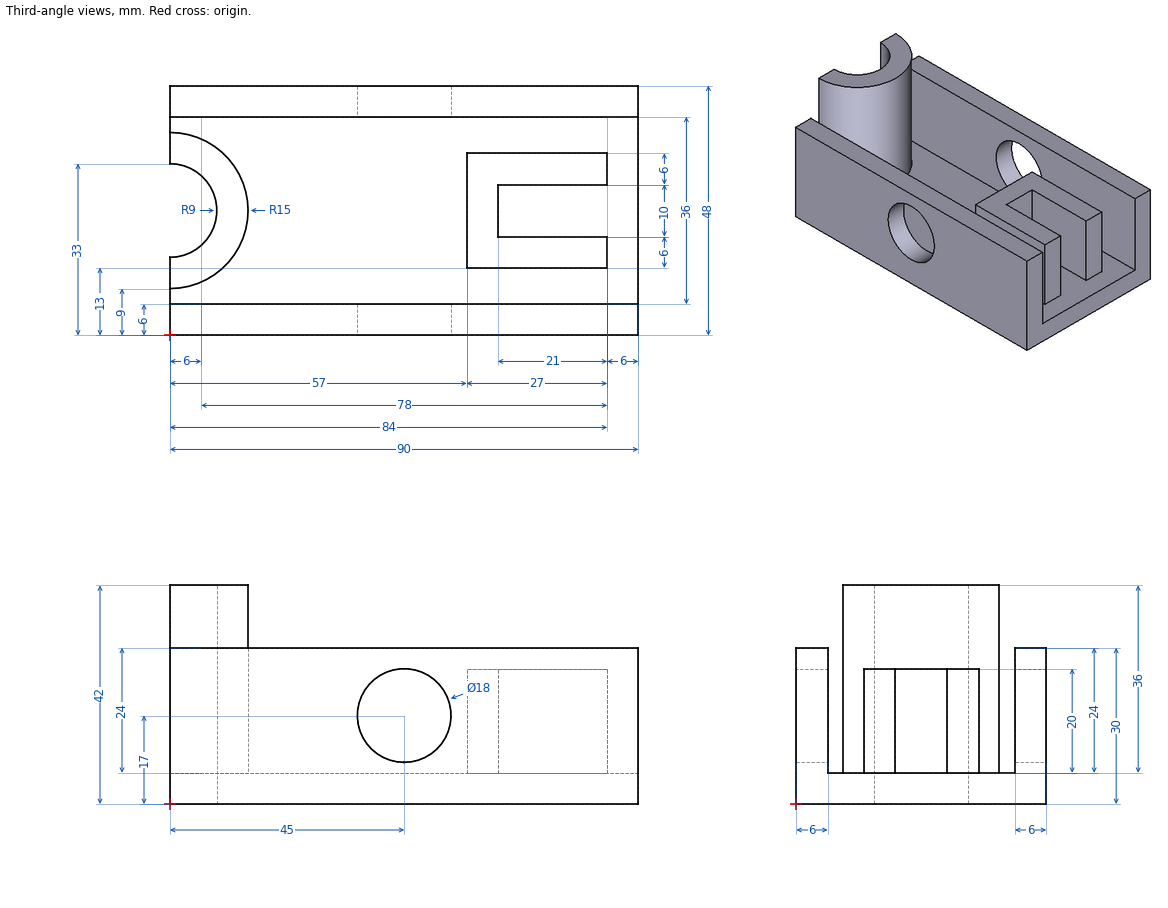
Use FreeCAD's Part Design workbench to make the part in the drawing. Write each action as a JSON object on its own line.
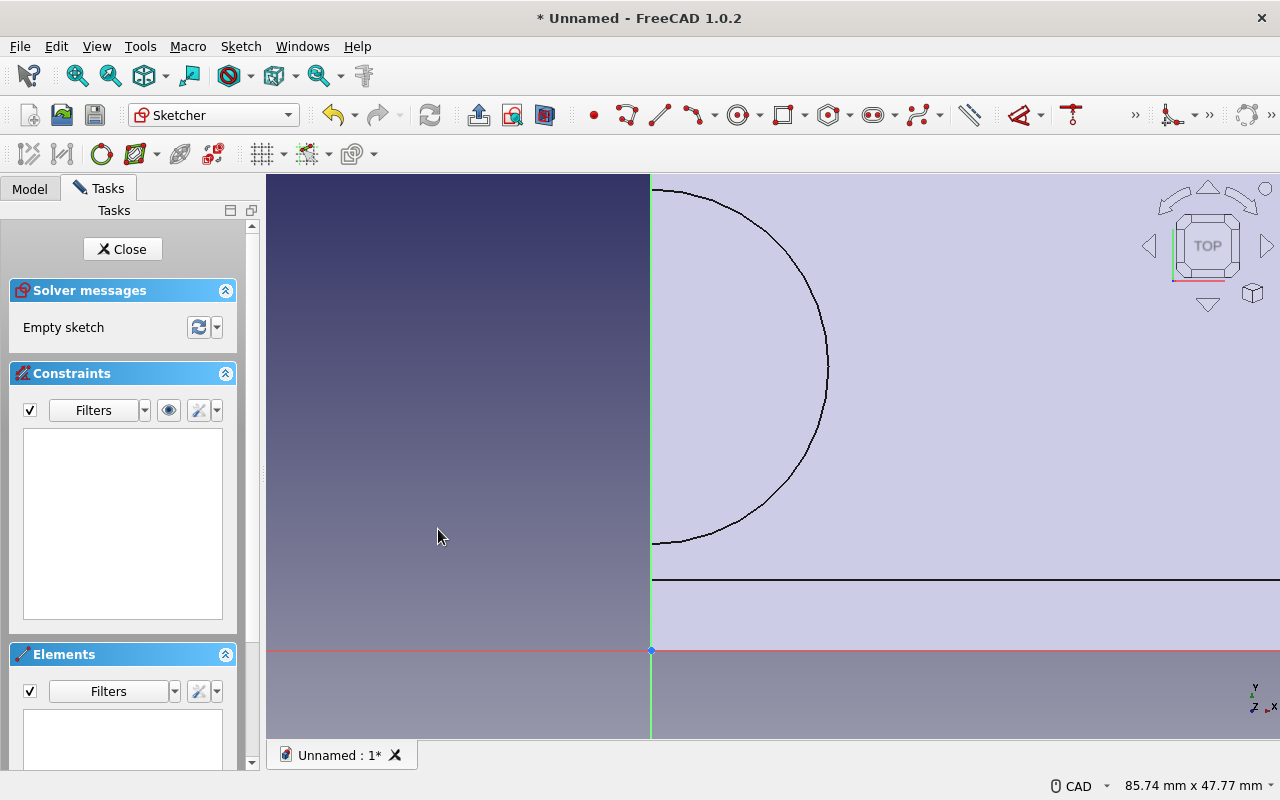
{"action": "left_click", "coordinate": [660, 116]}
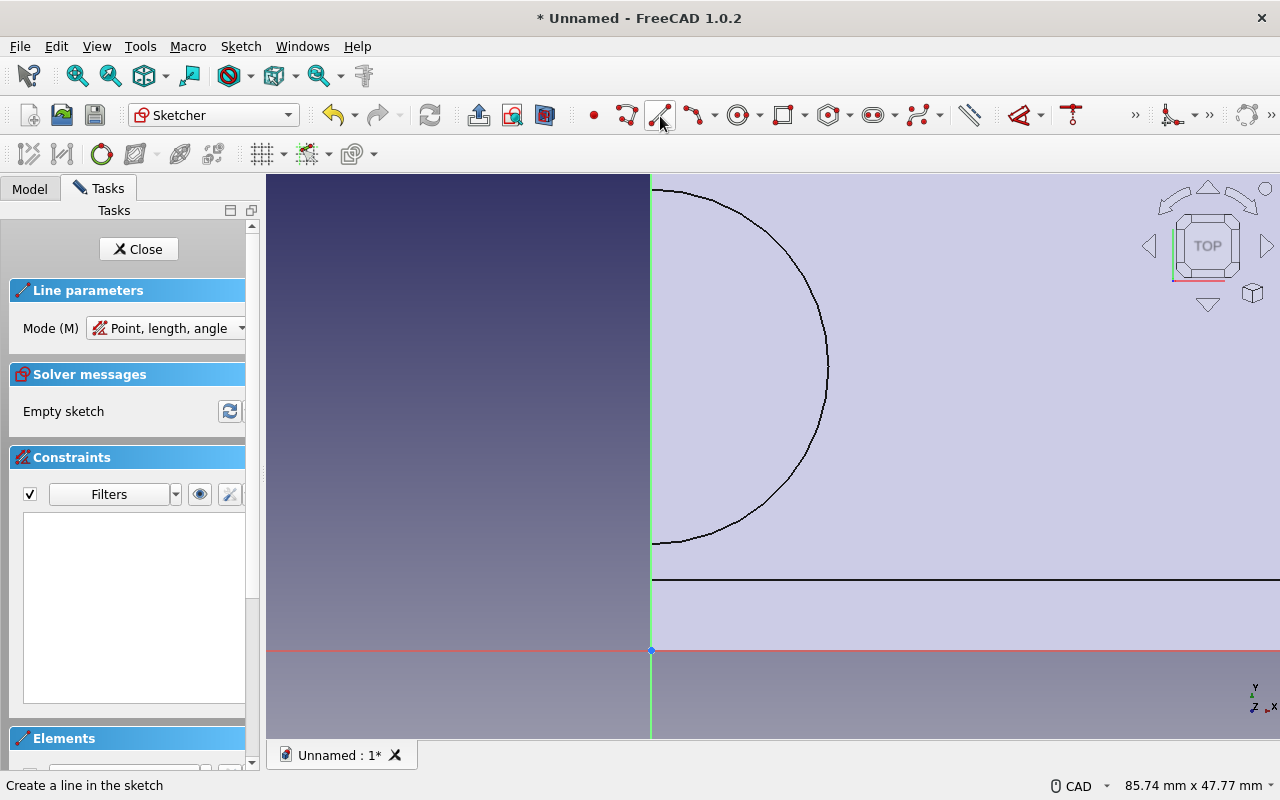
{"action": "left_click", "coordinate": [651, 260]}
{"action": "left_click", "coordinate": [660, 473]}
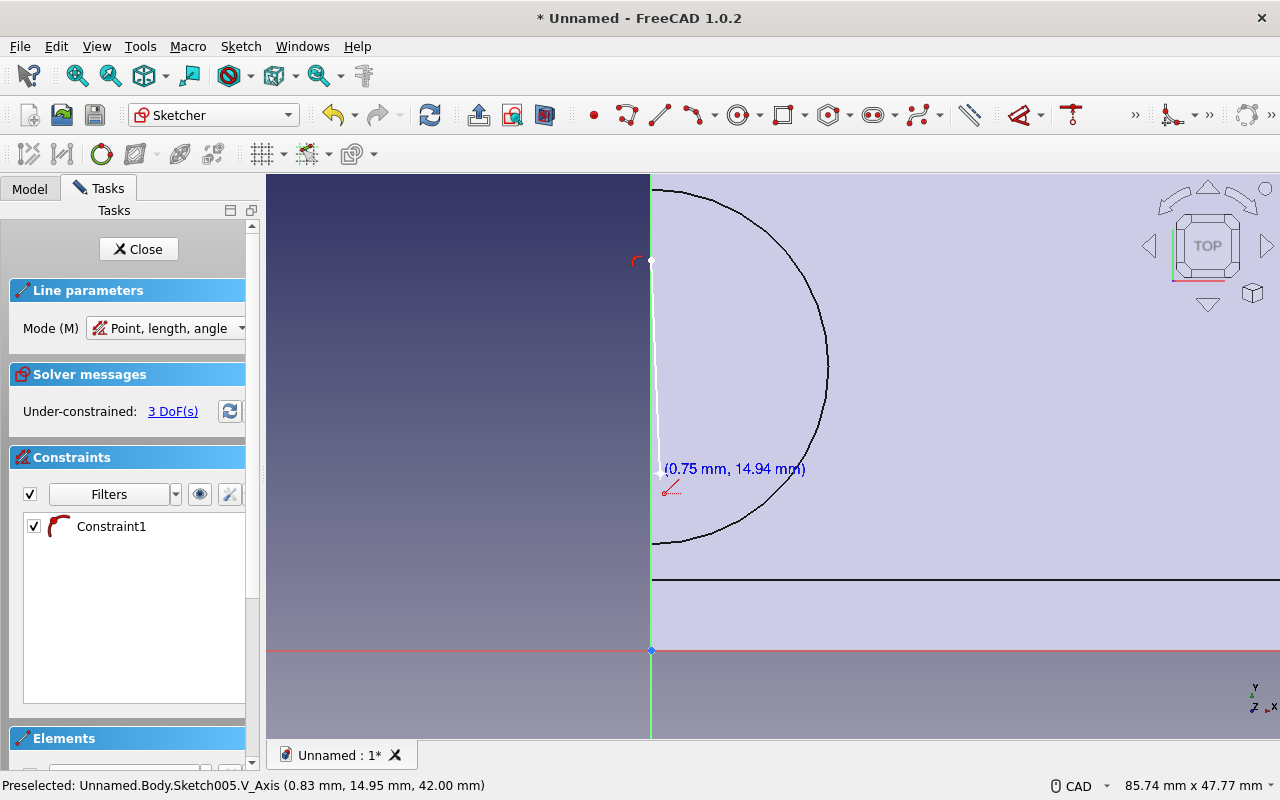
{"action": "key", "text": "g 3 a"}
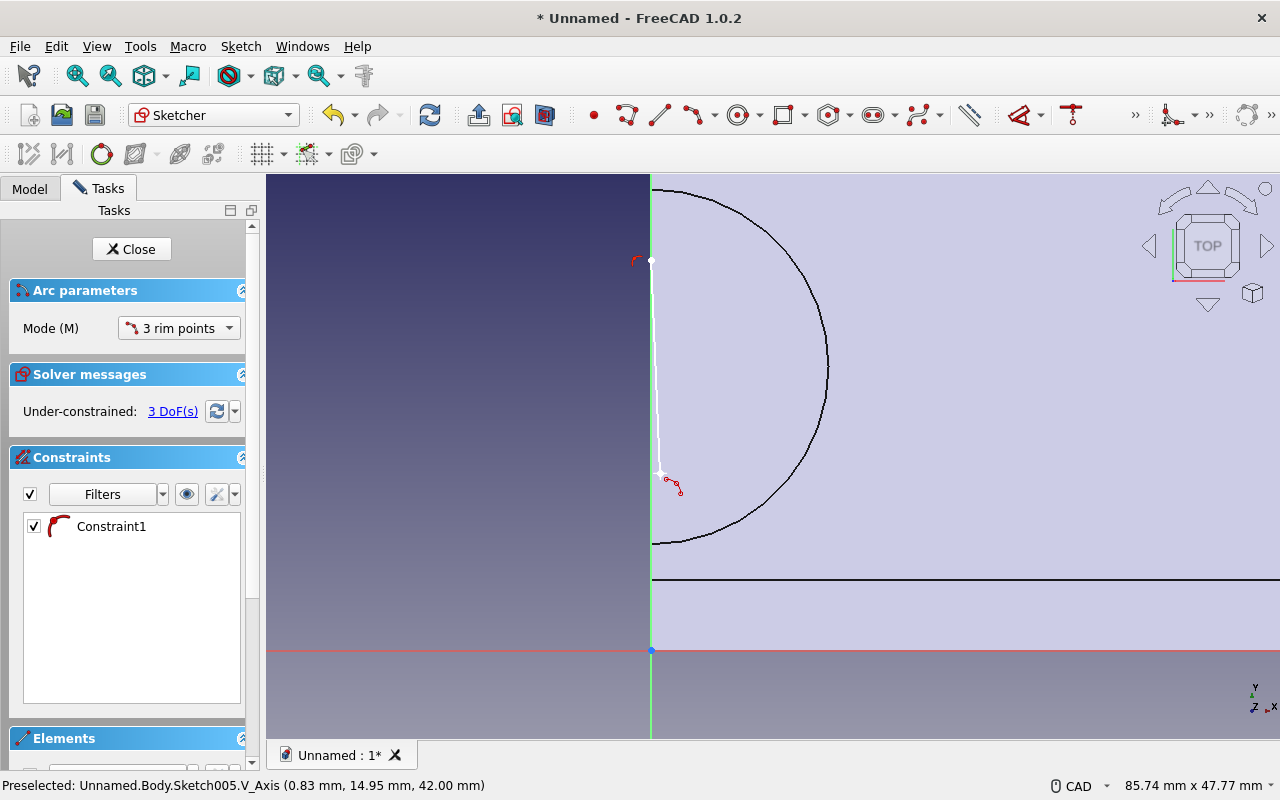
{"action": "left_click", "coordinate": [660, 474]}
{"action": "left_click", "coordinate": [651, 261]}
{"action": "left_click", "coordinate": [758, 367]}
{"action": "key", "text": "Escape"}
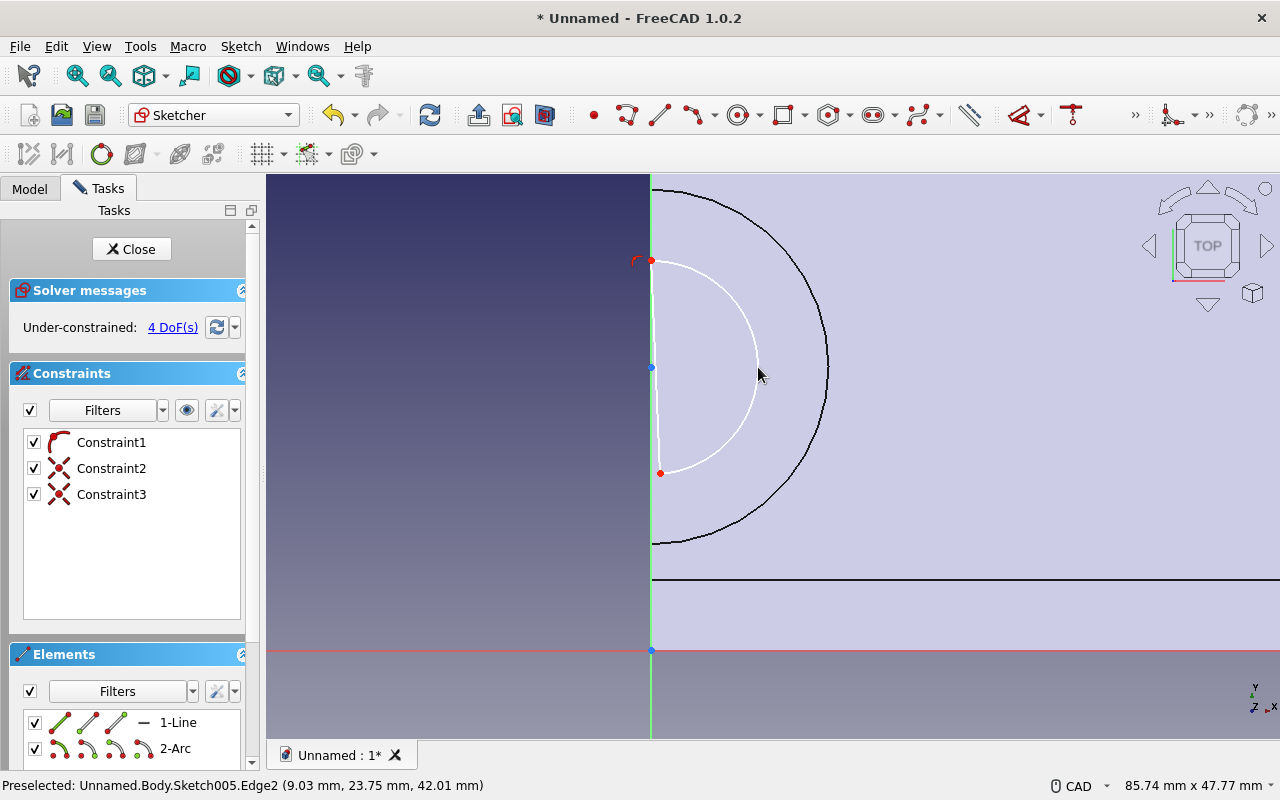
{"action": "left_click", "coordinate": [654, 325]}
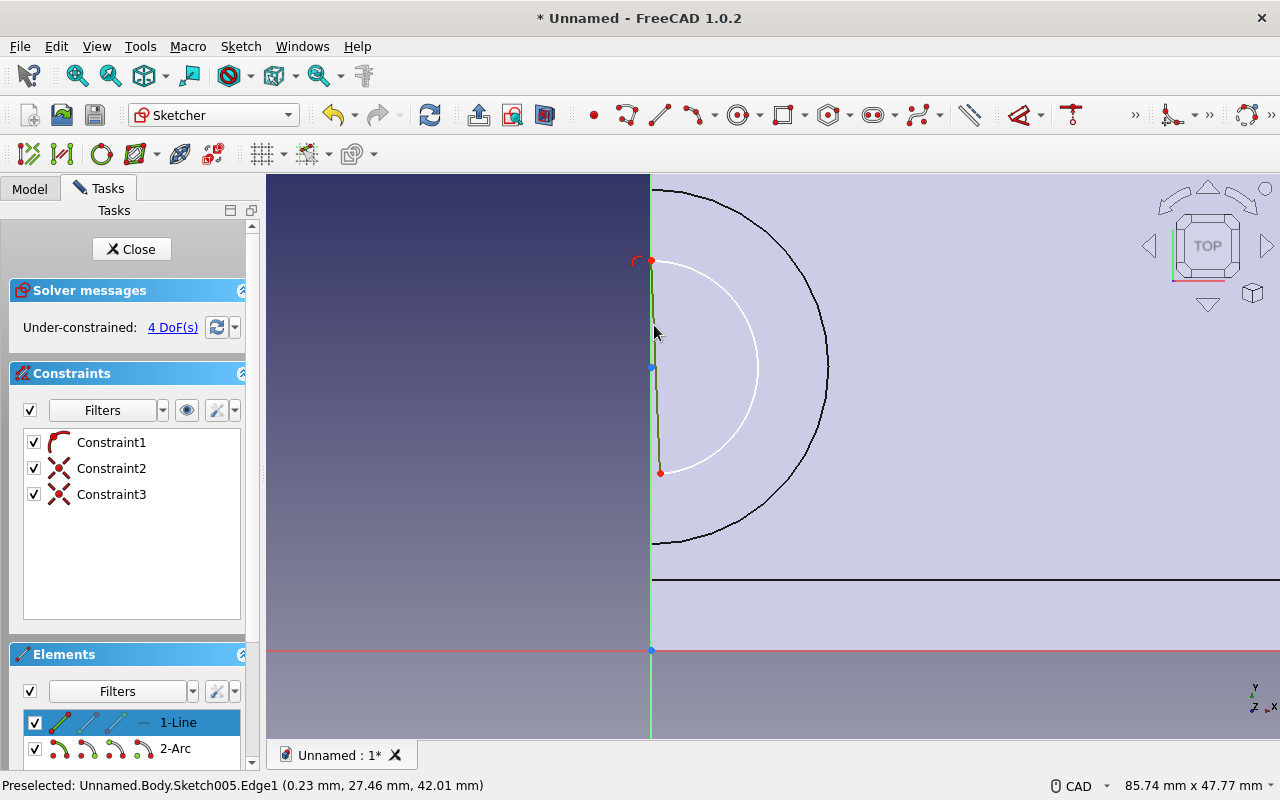
{"action": "key", "text": "v"}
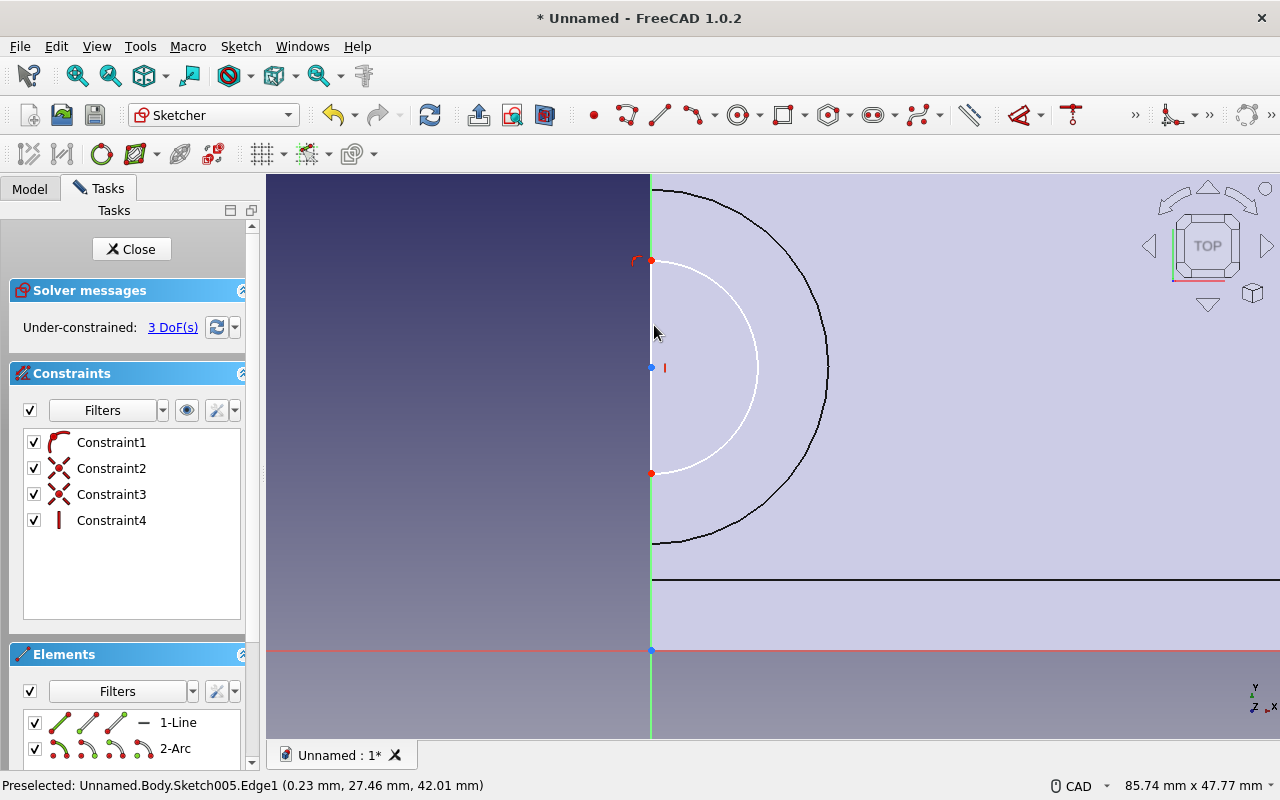
{"action": "left_click", "coordinate": [651, 368]}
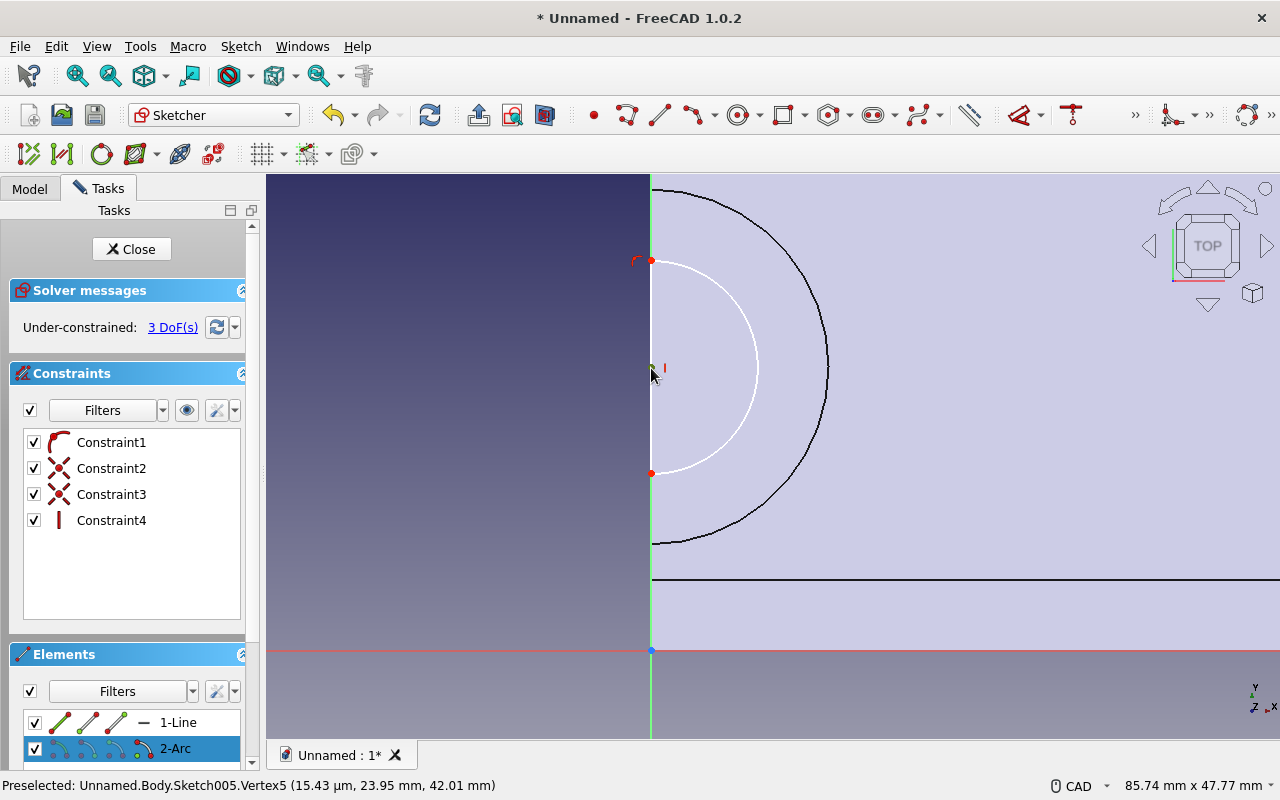
{"action": "left_click", "coordinate": [651, 602]}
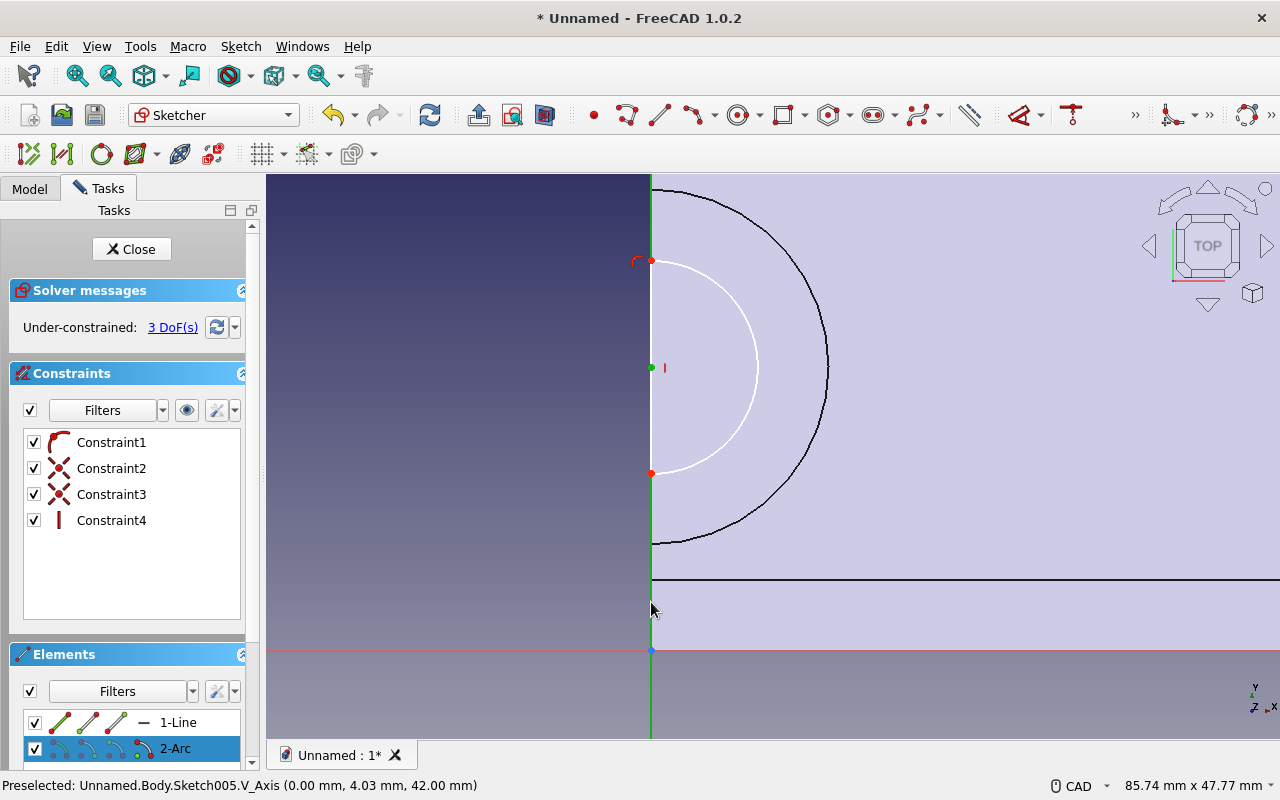
{"action": "key", "text": "c"}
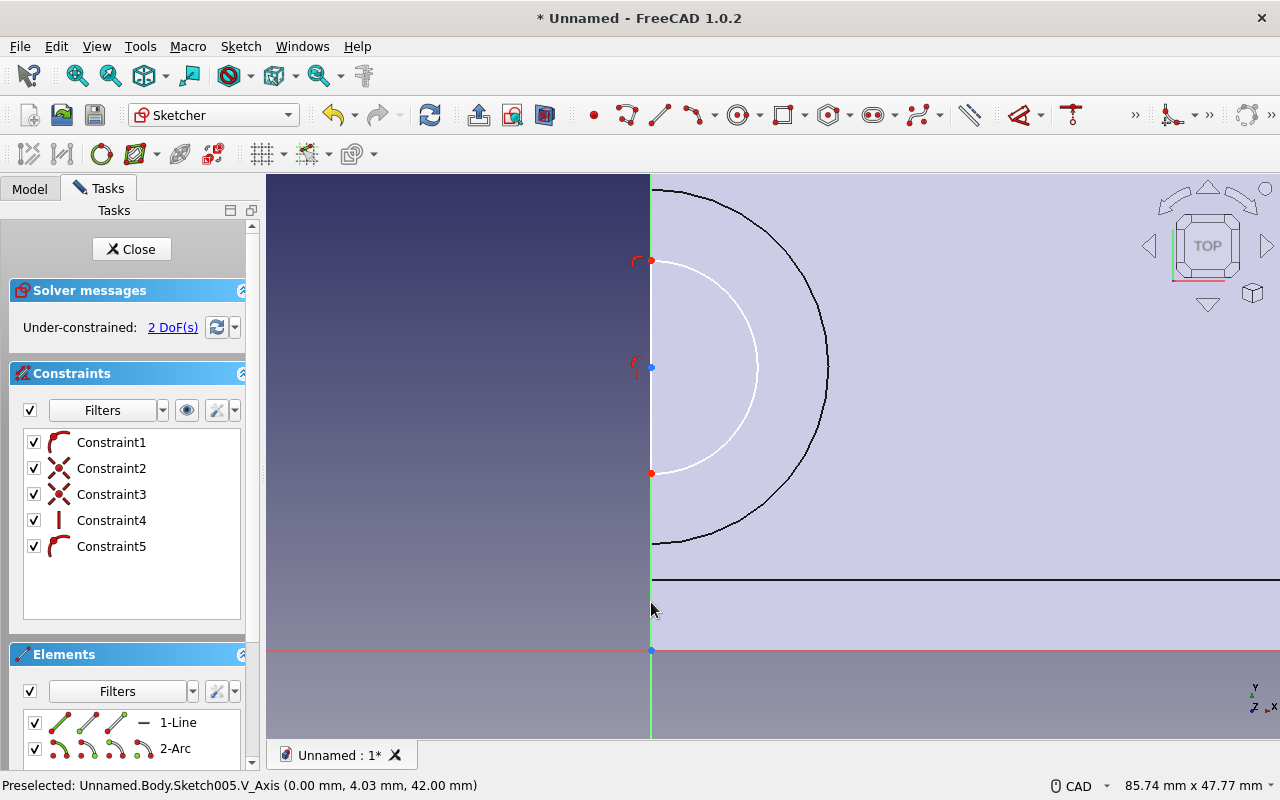
{"action": "key", "text": "d"}